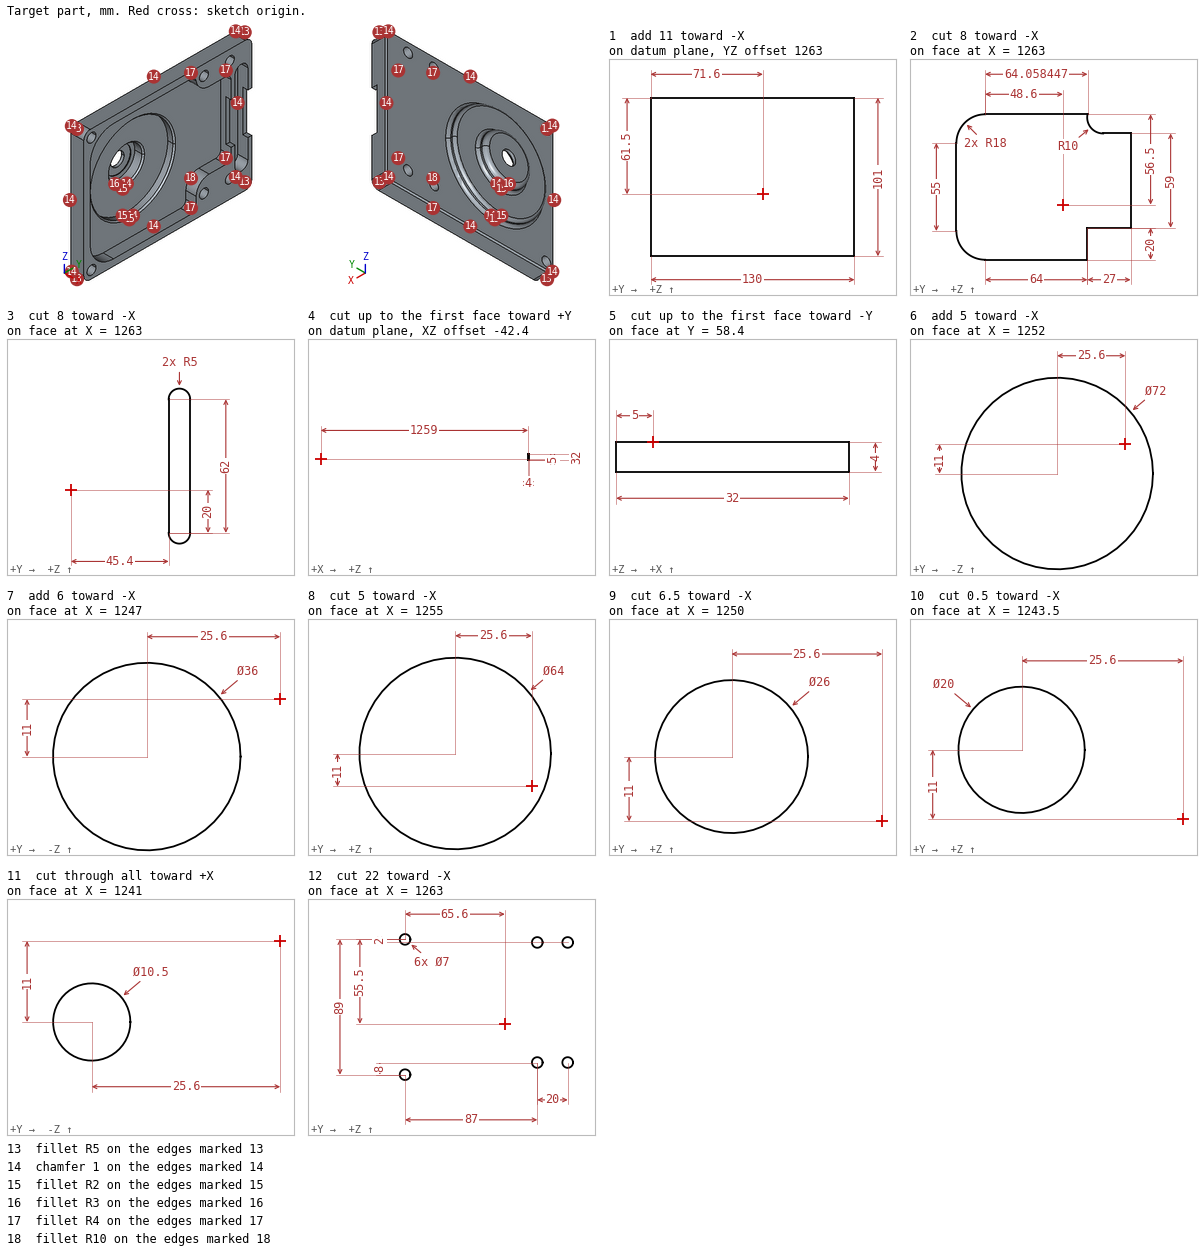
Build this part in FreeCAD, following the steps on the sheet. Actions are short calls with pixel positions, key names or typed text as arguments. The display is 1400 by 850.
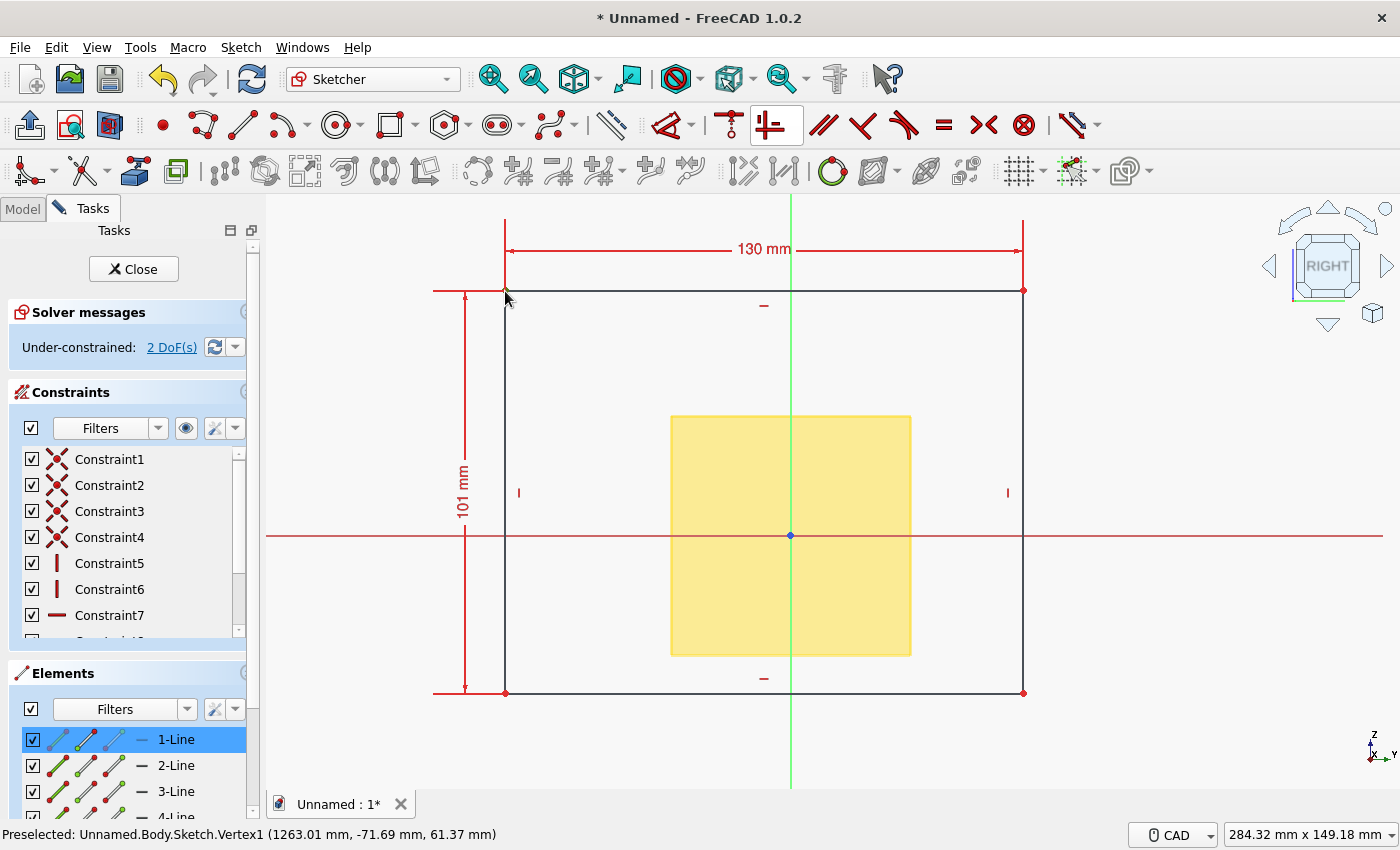
click(694, 126)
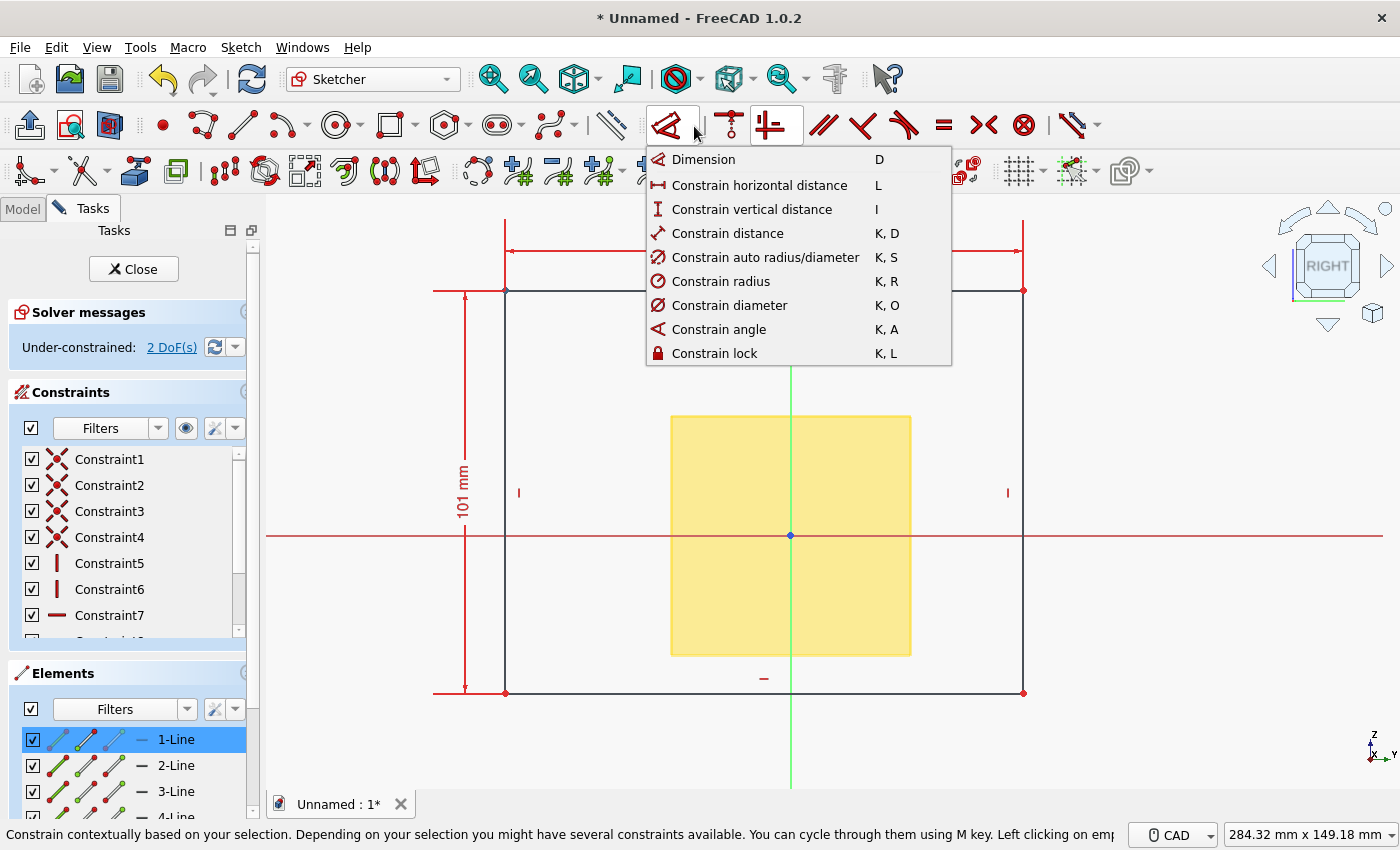
click(799, 185)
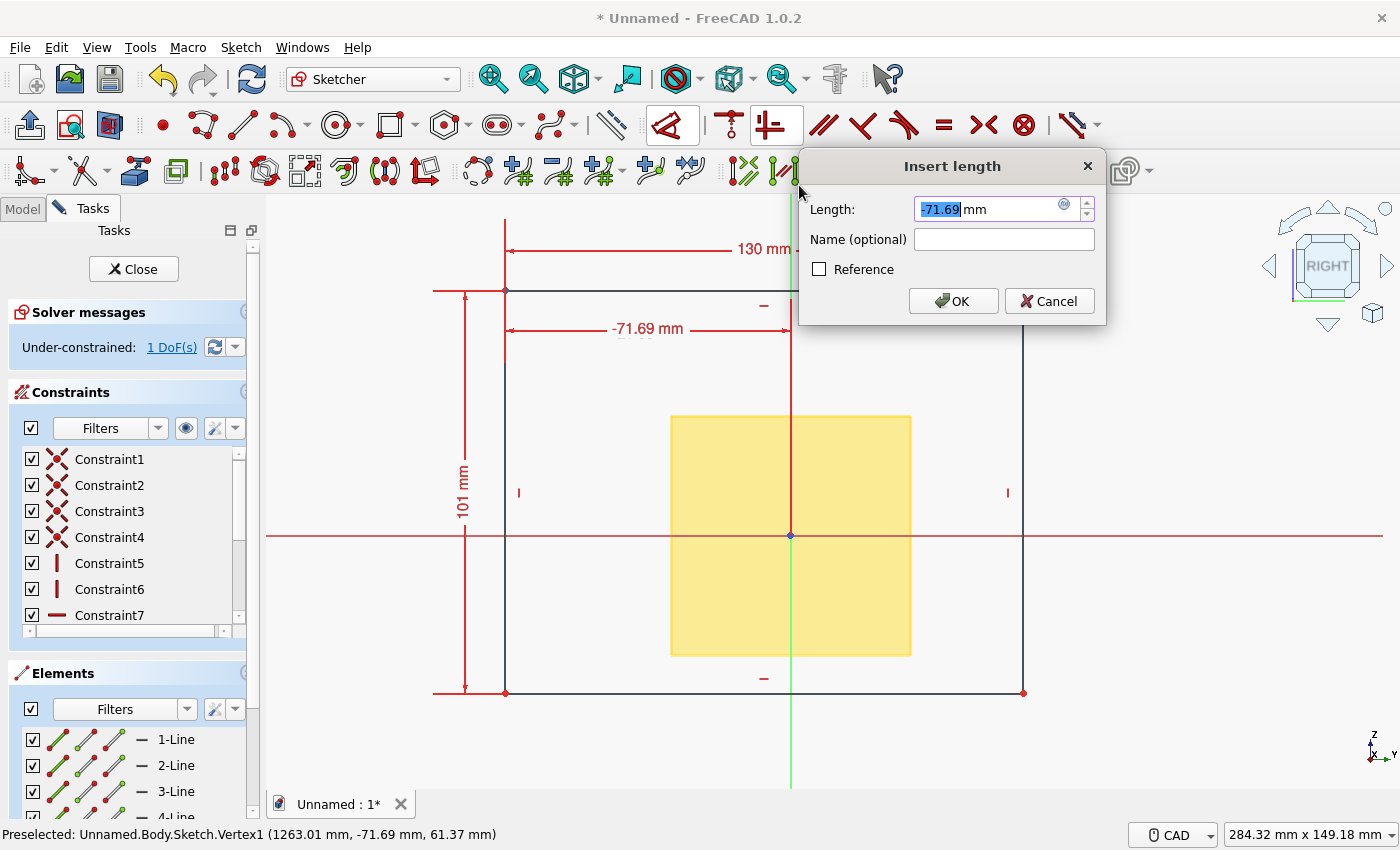
text(-71.6)
key(Return)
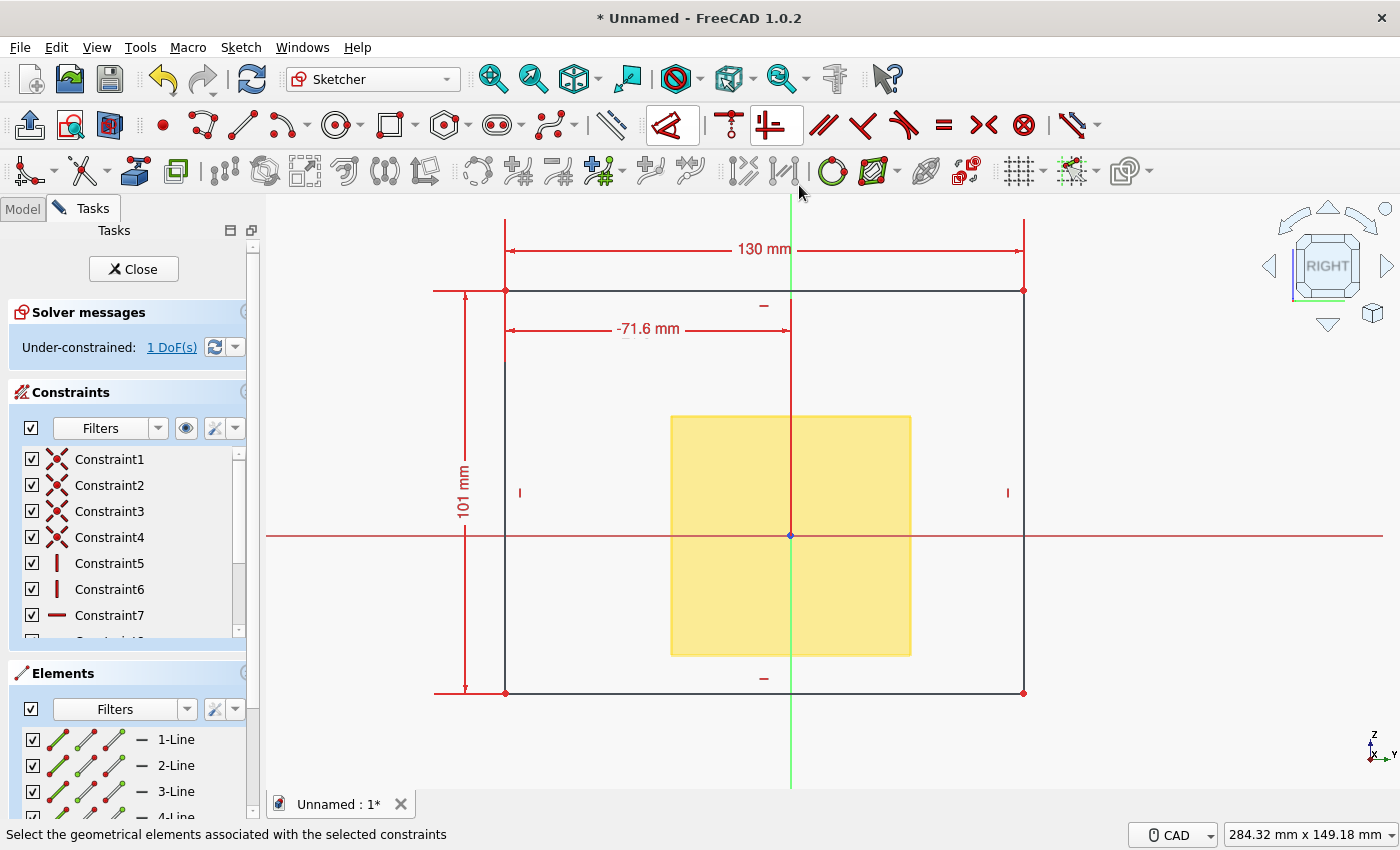
click(505, 291)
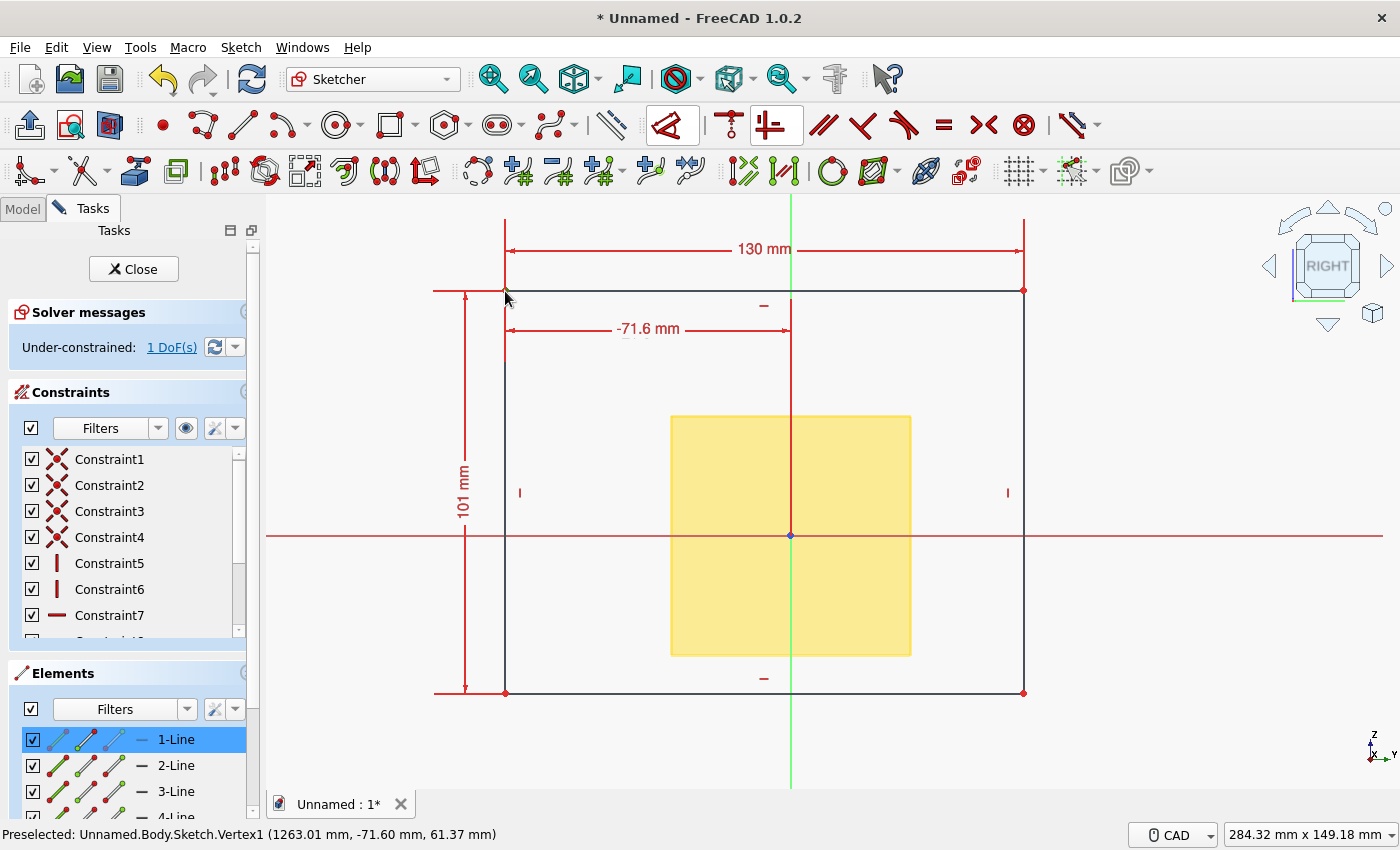
key(i)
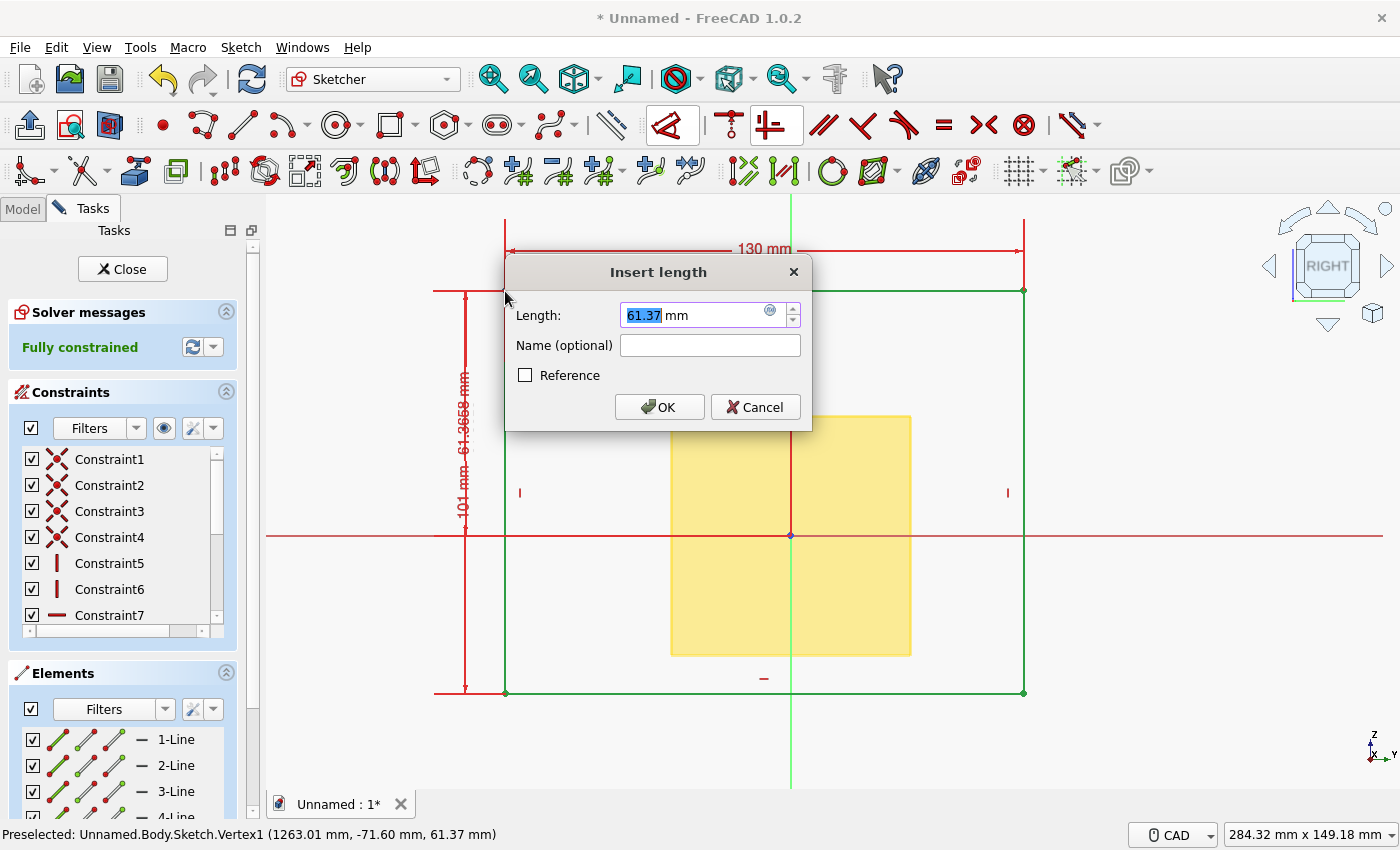
text(61.5)
key(Return)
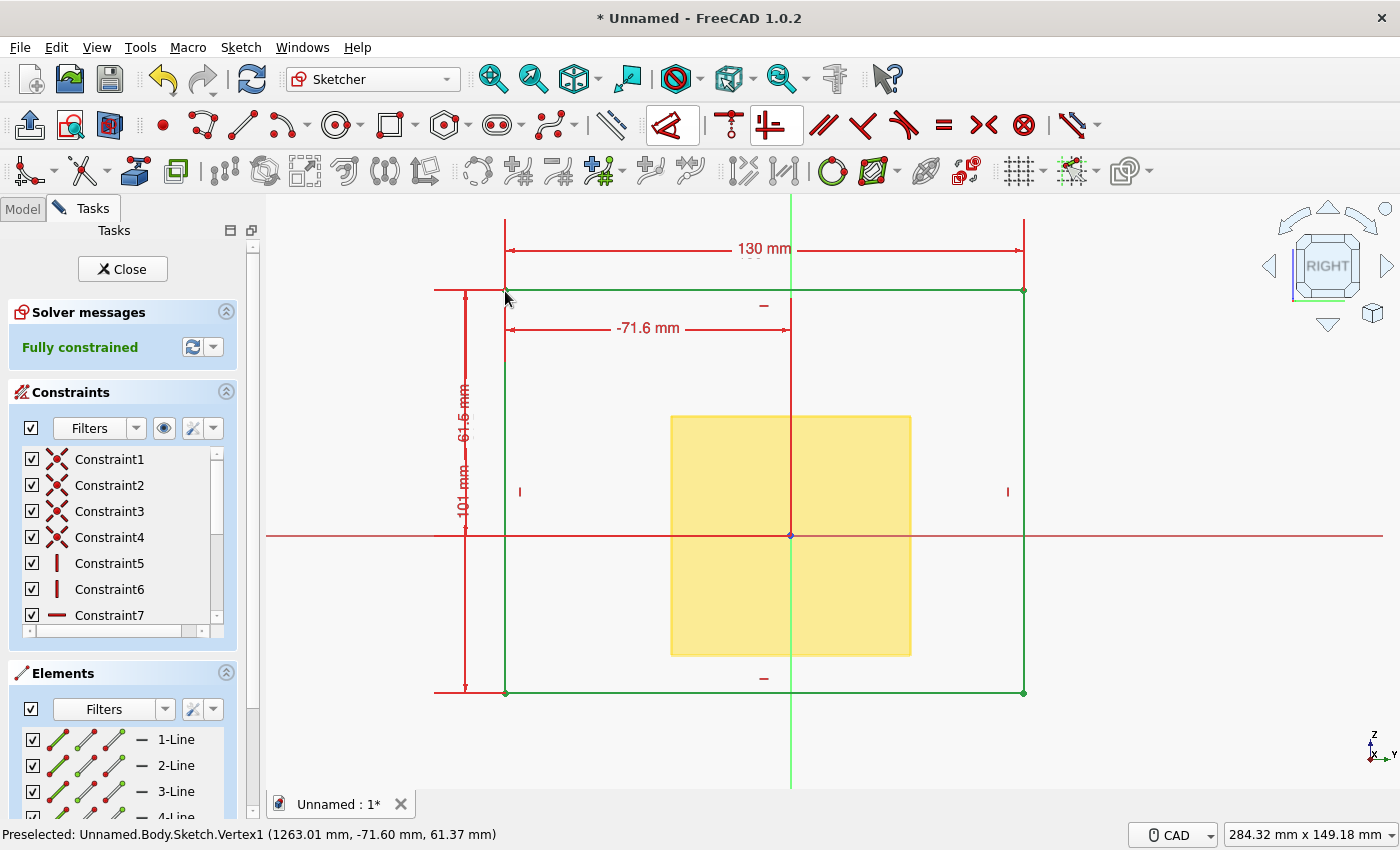
click(123, 269)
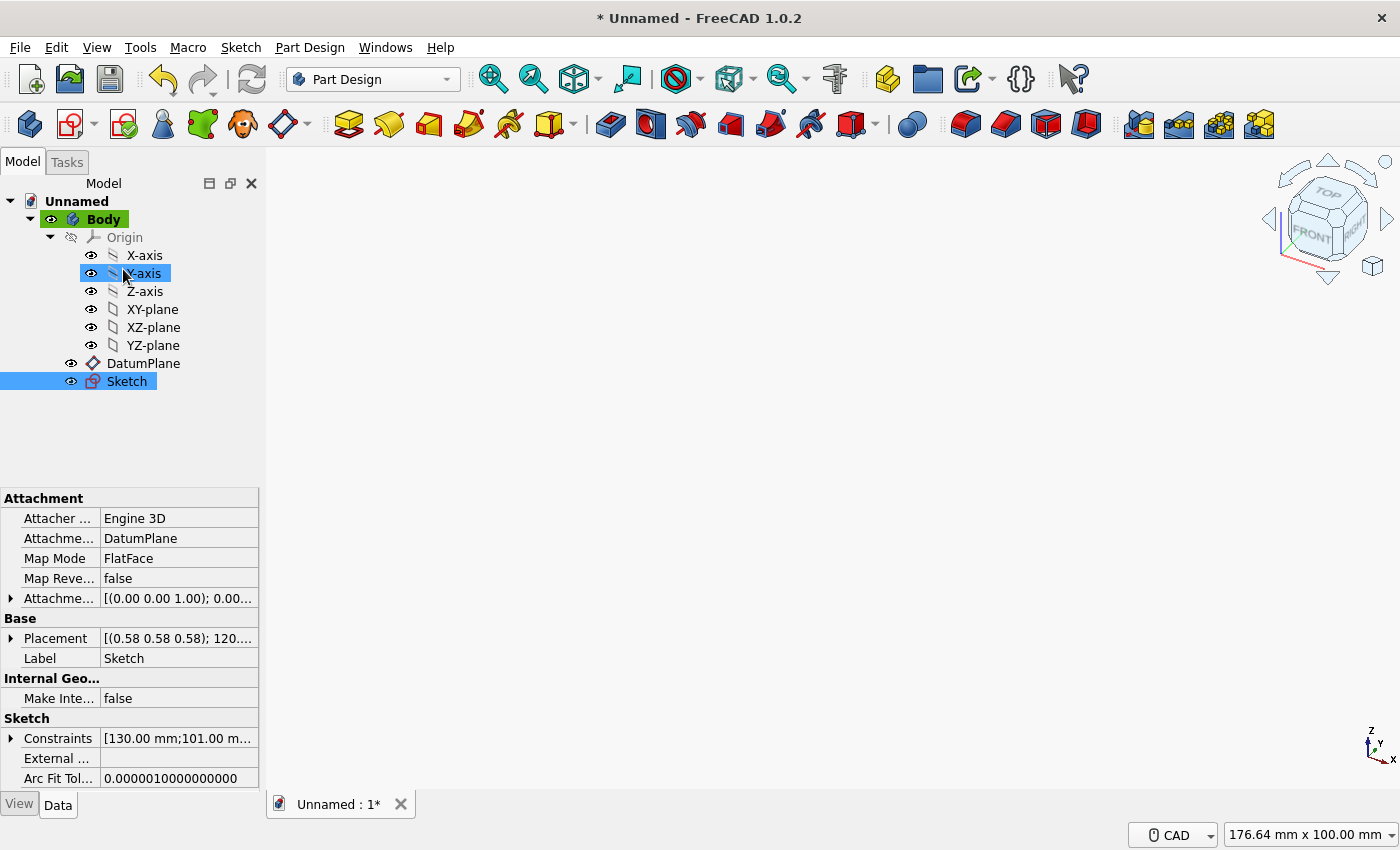
click(350, 124)